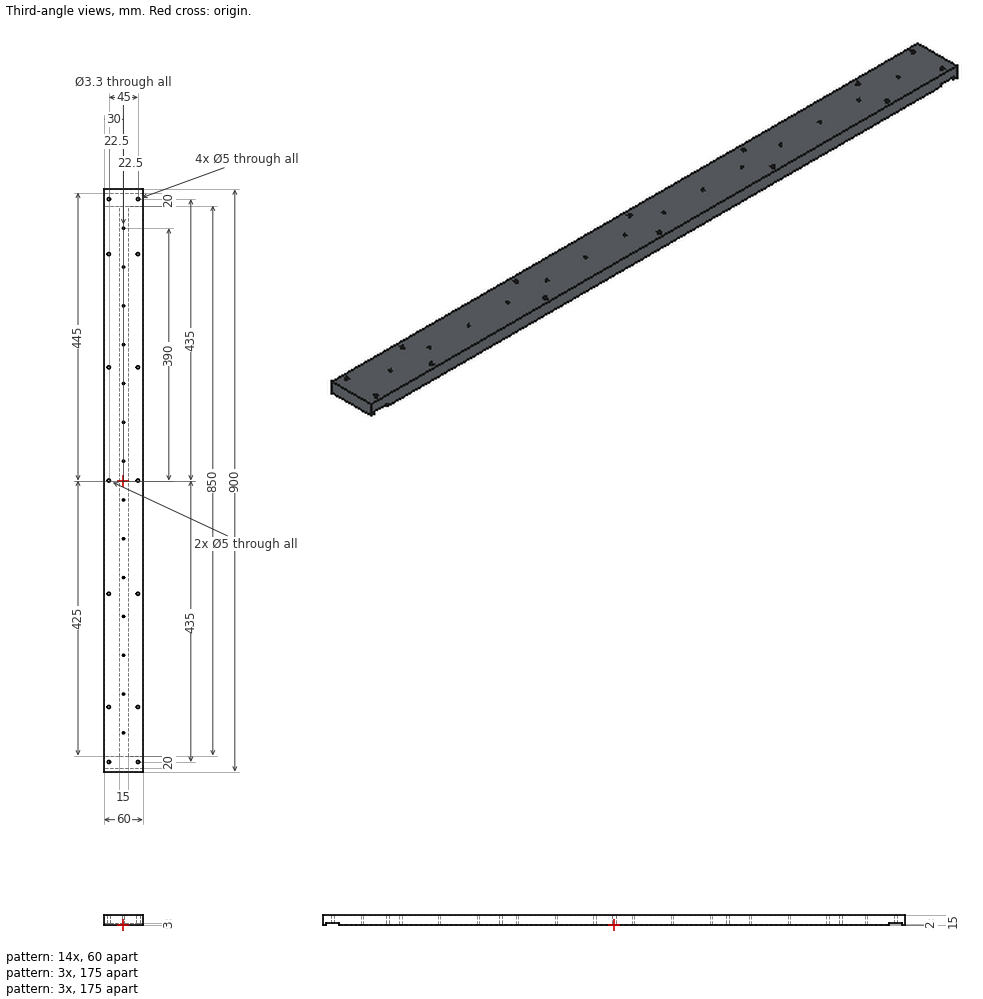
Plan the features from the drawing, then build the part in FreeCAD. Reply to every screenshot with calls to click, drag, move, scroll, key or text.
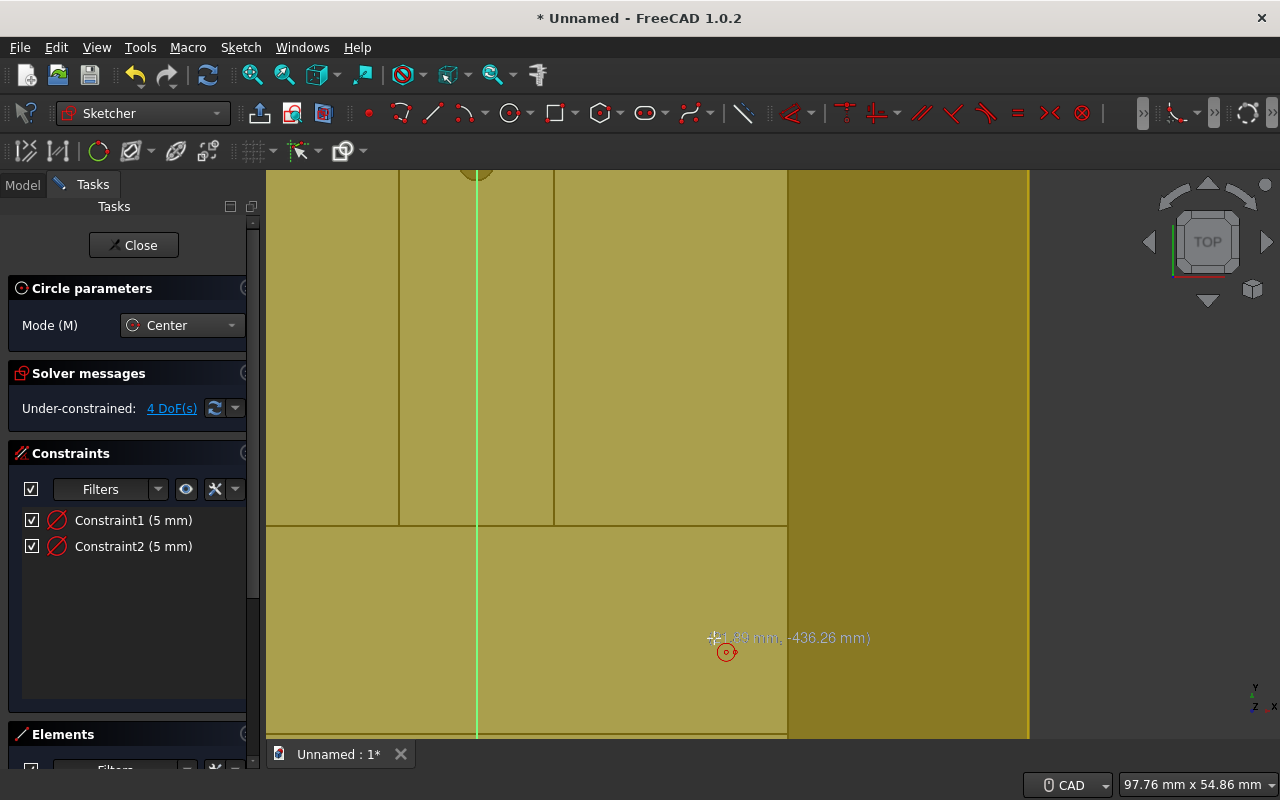
scroll(716, 682, down, 15)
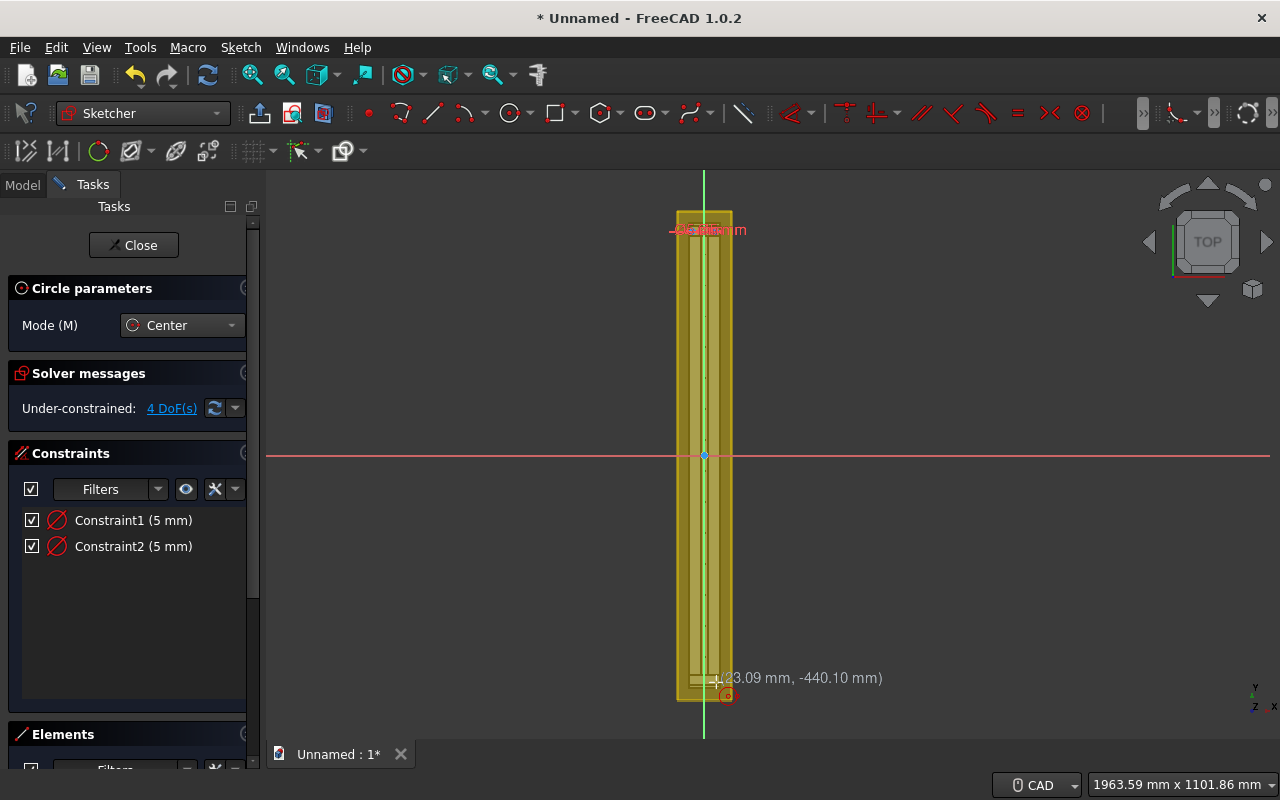
scroll(716, 680, up, 2)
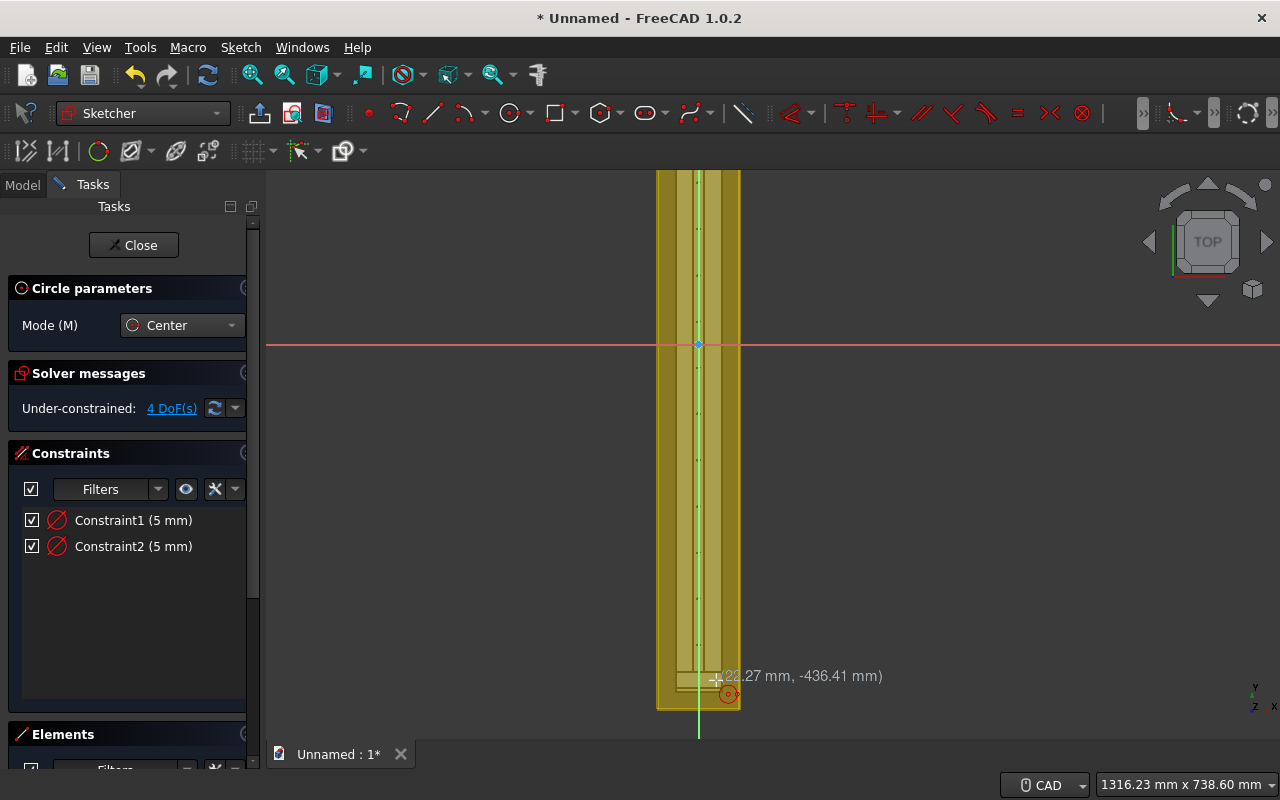
click(716, 680)
move(717, 679)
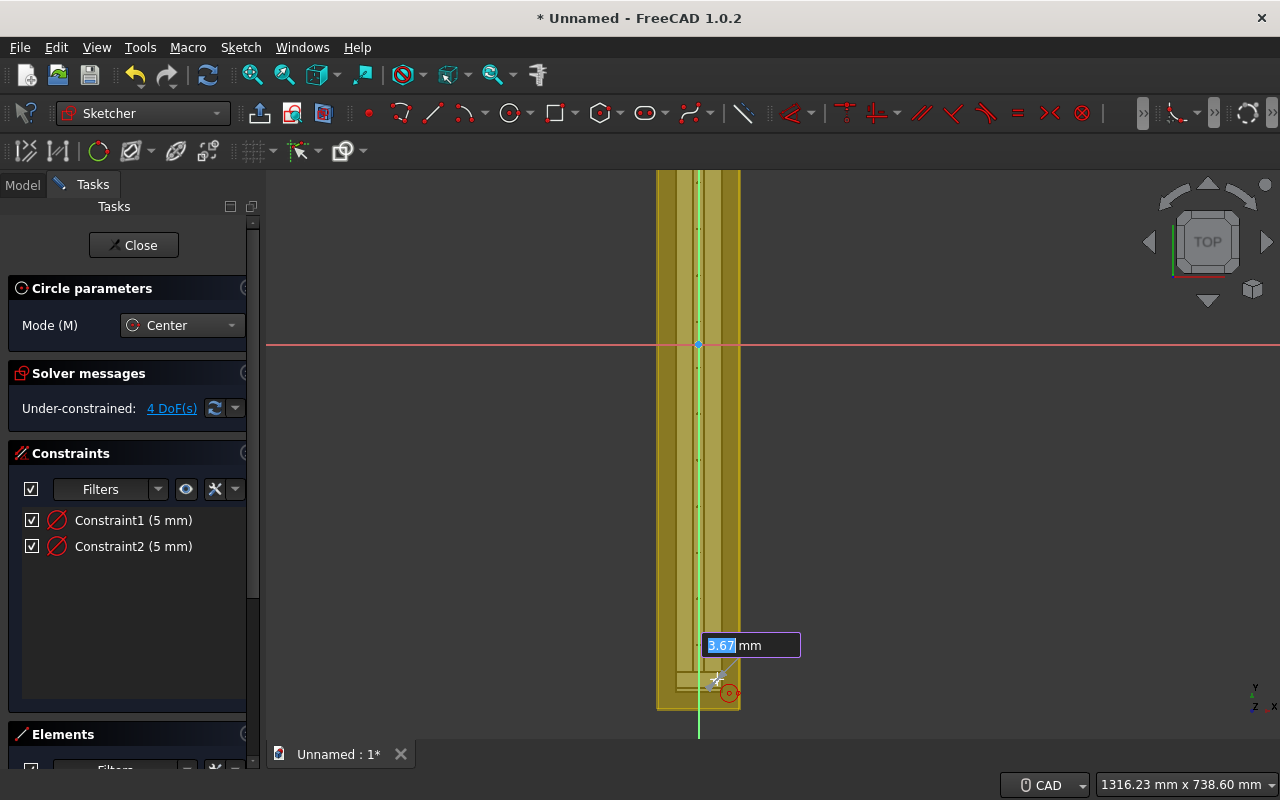
text(5)
key(Return)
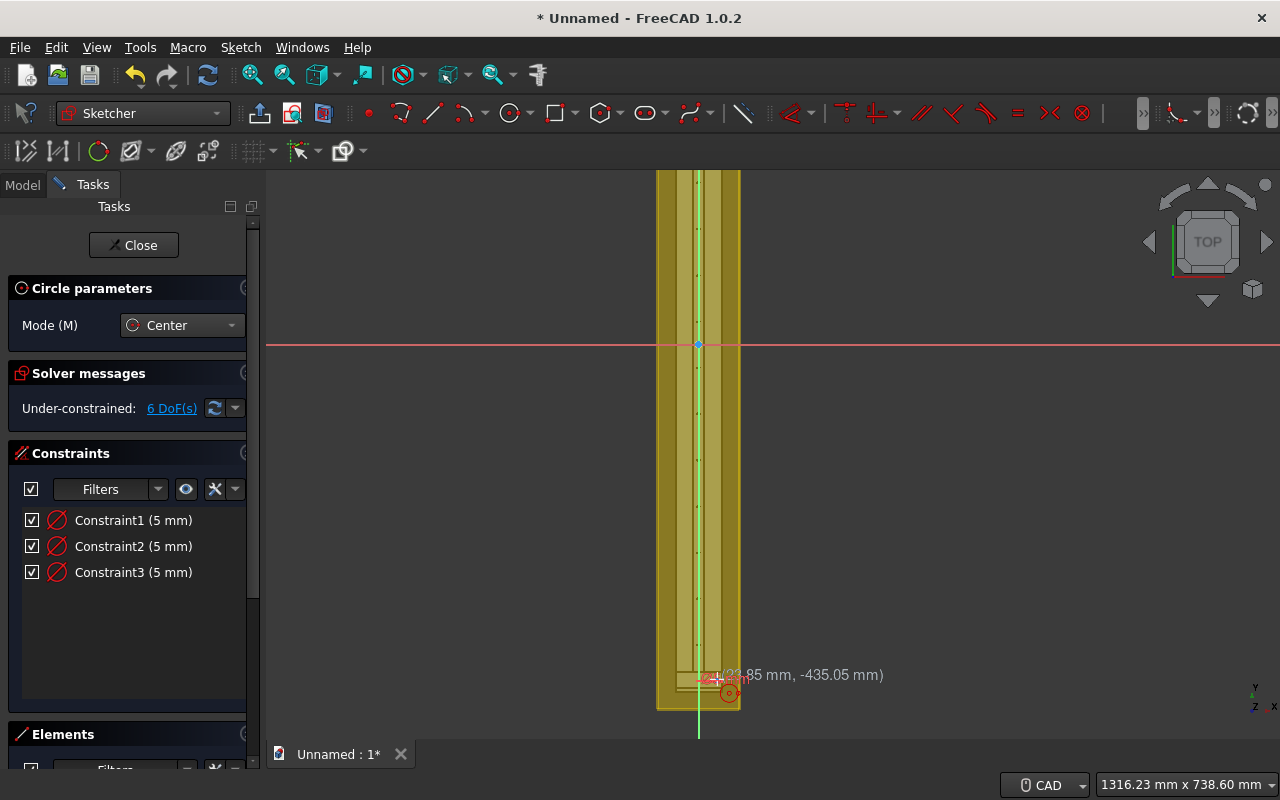
scroll(681, 680, up, 13)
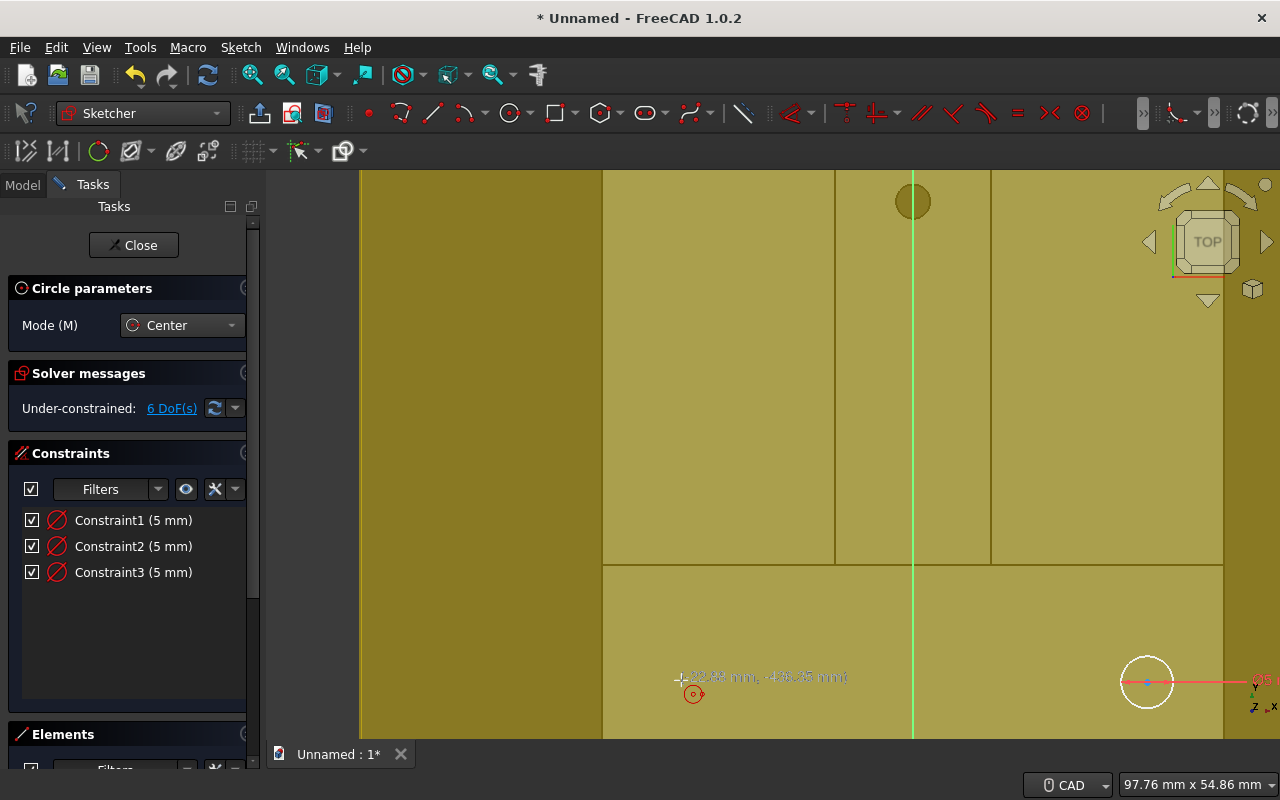
scroll(694, 680, down, 15)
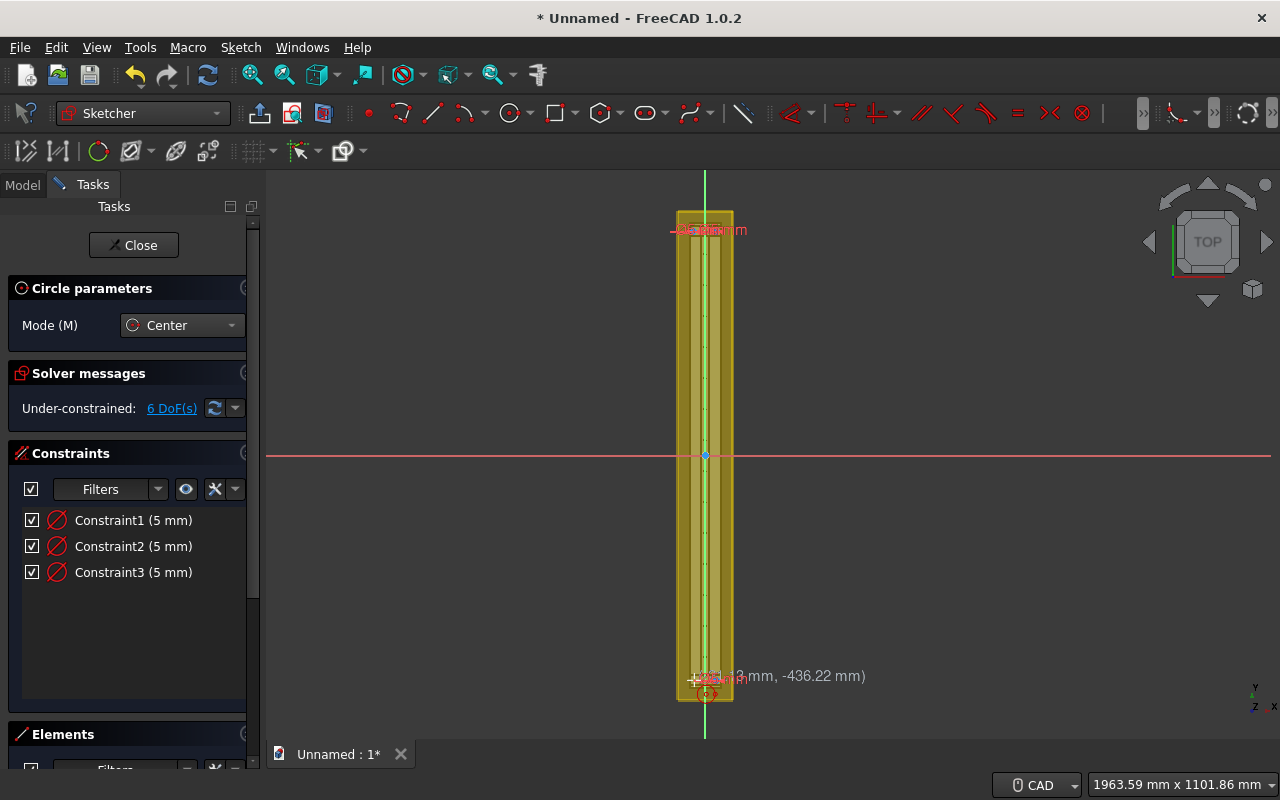
scroll(694, 680, up, 2)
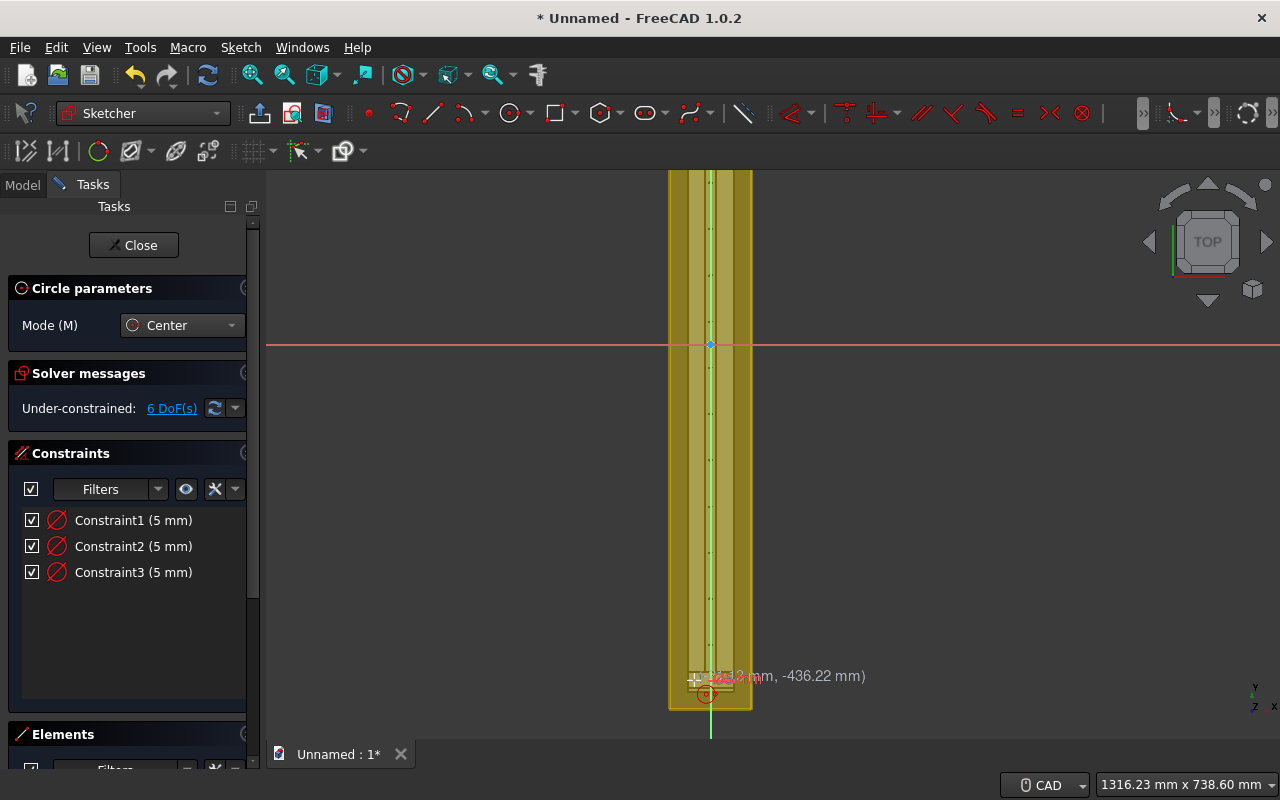
click(693, 680)
move(695, 679)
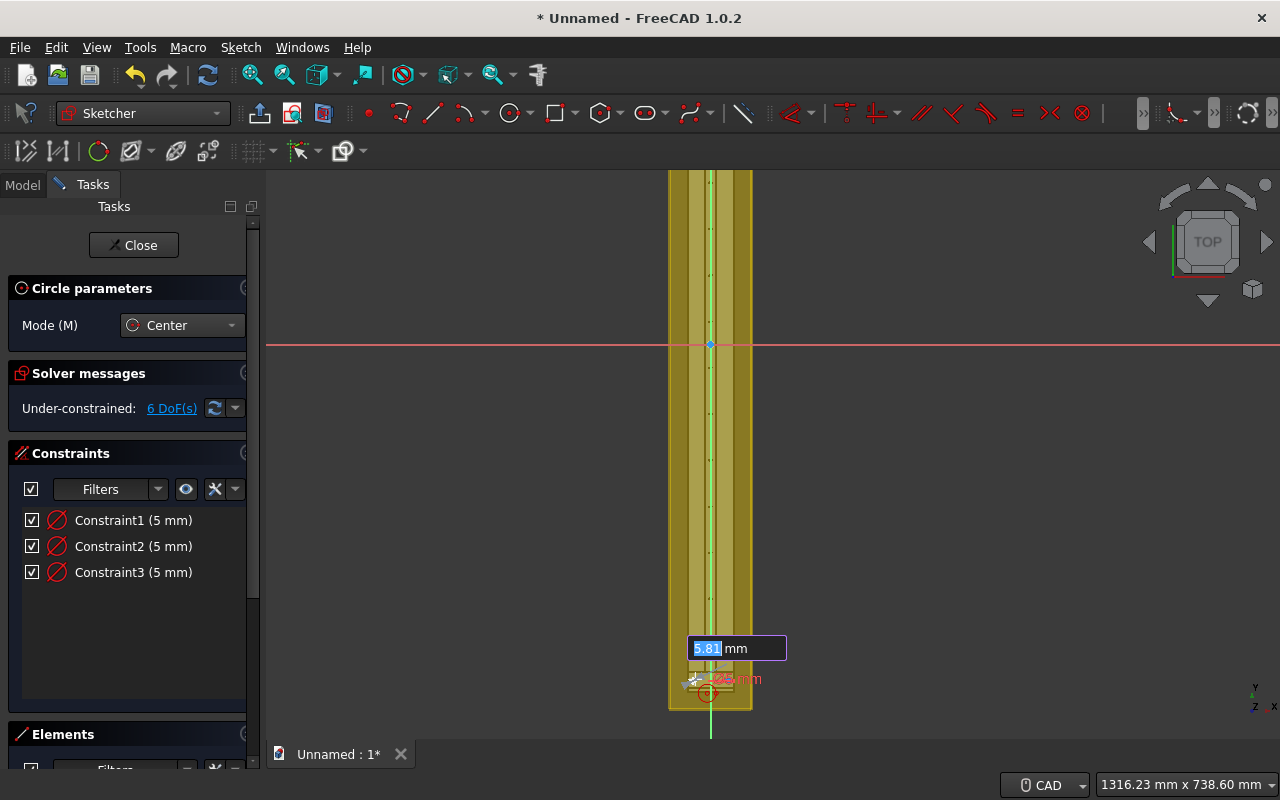
text(5)
key(Return)
key(Escape)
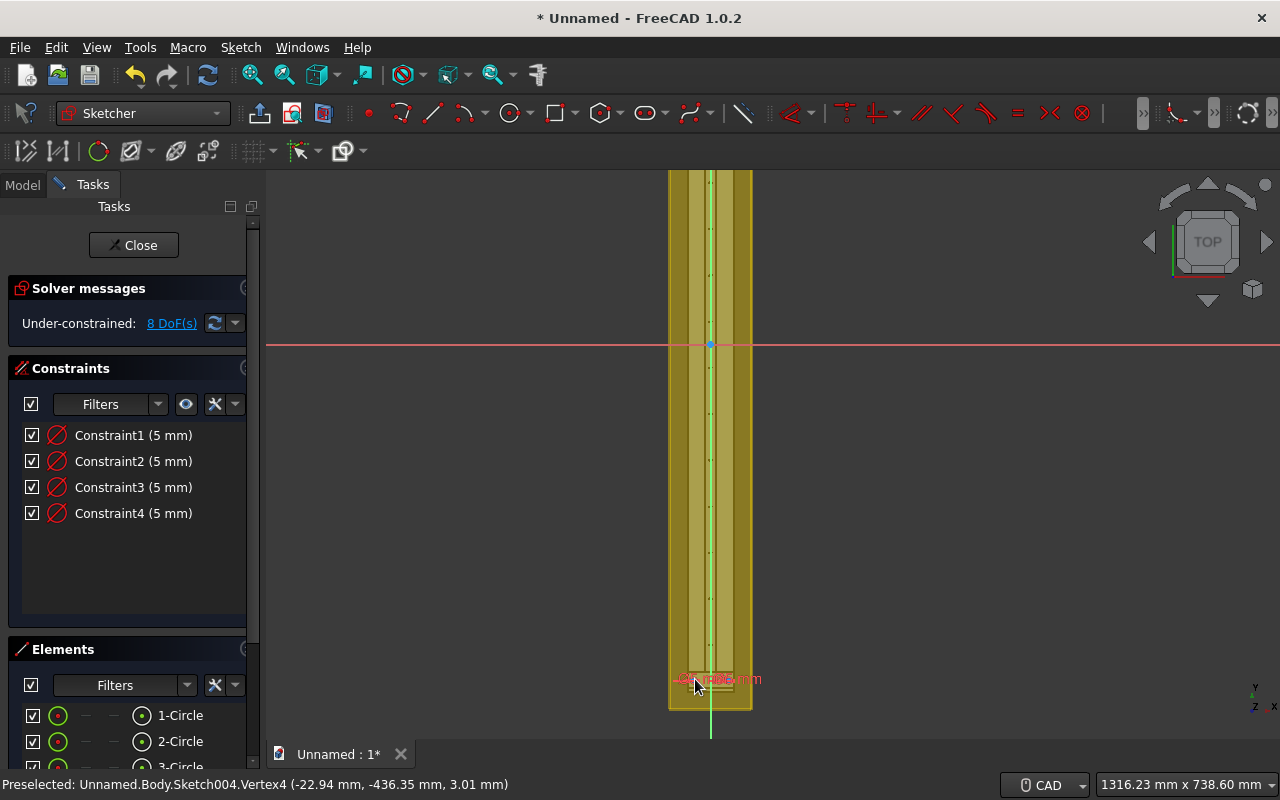
scroll(697, 588, down, 3)